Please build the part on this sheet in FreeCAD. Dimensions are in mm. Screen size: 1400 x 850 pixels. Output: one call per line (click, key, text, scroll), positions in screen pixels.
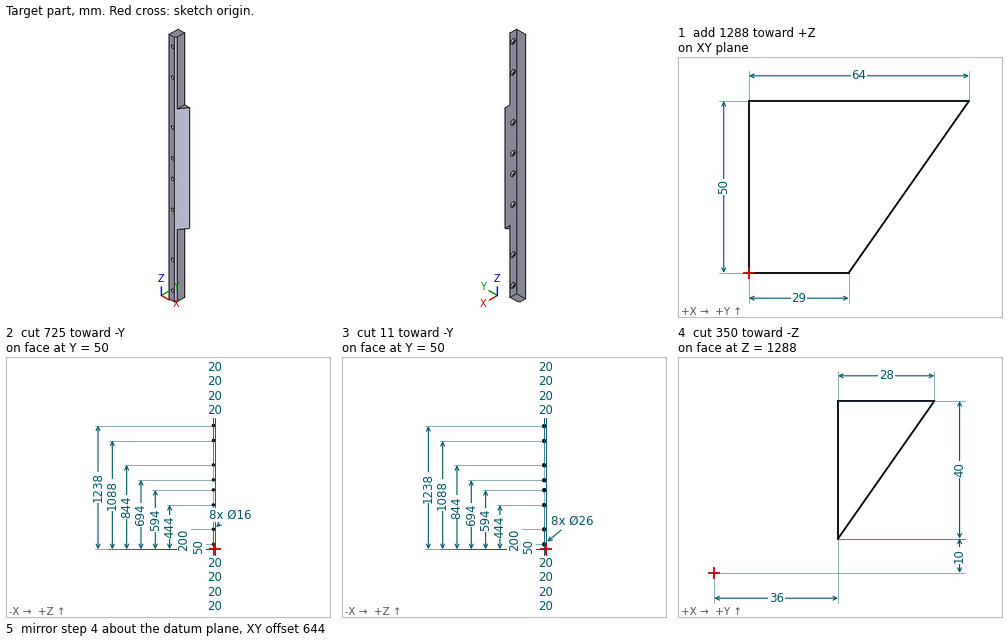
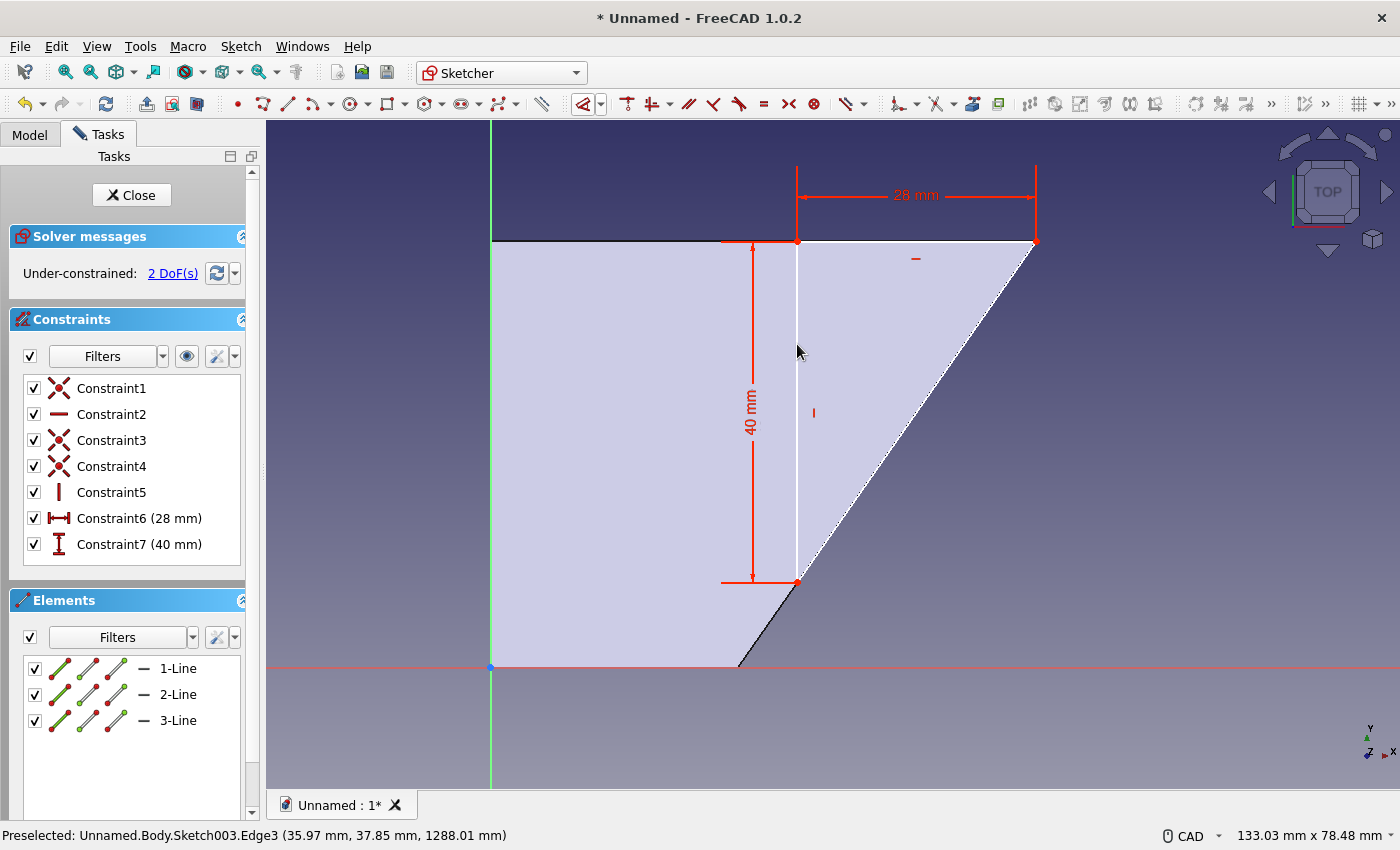
click(797, 583)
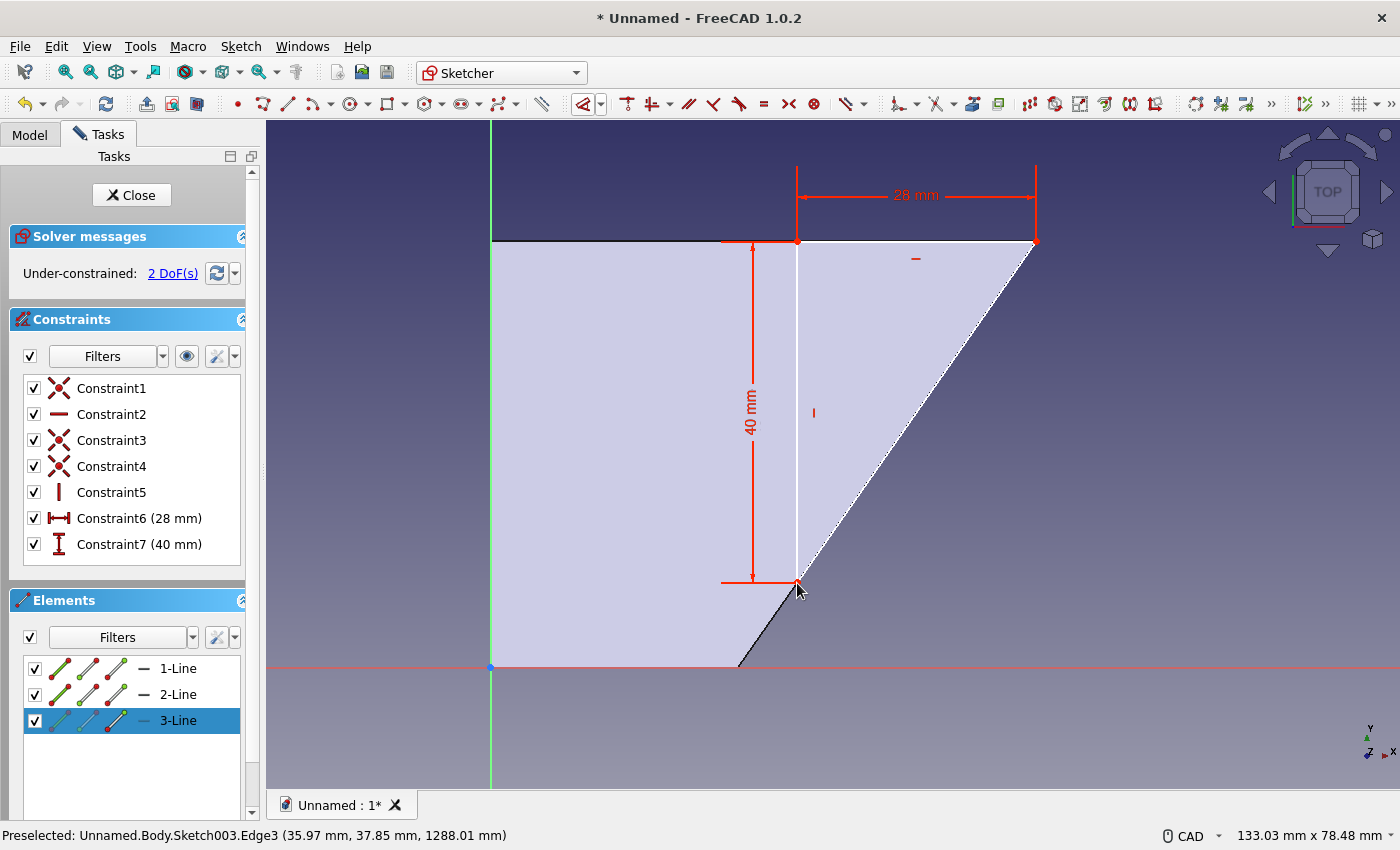
key(l)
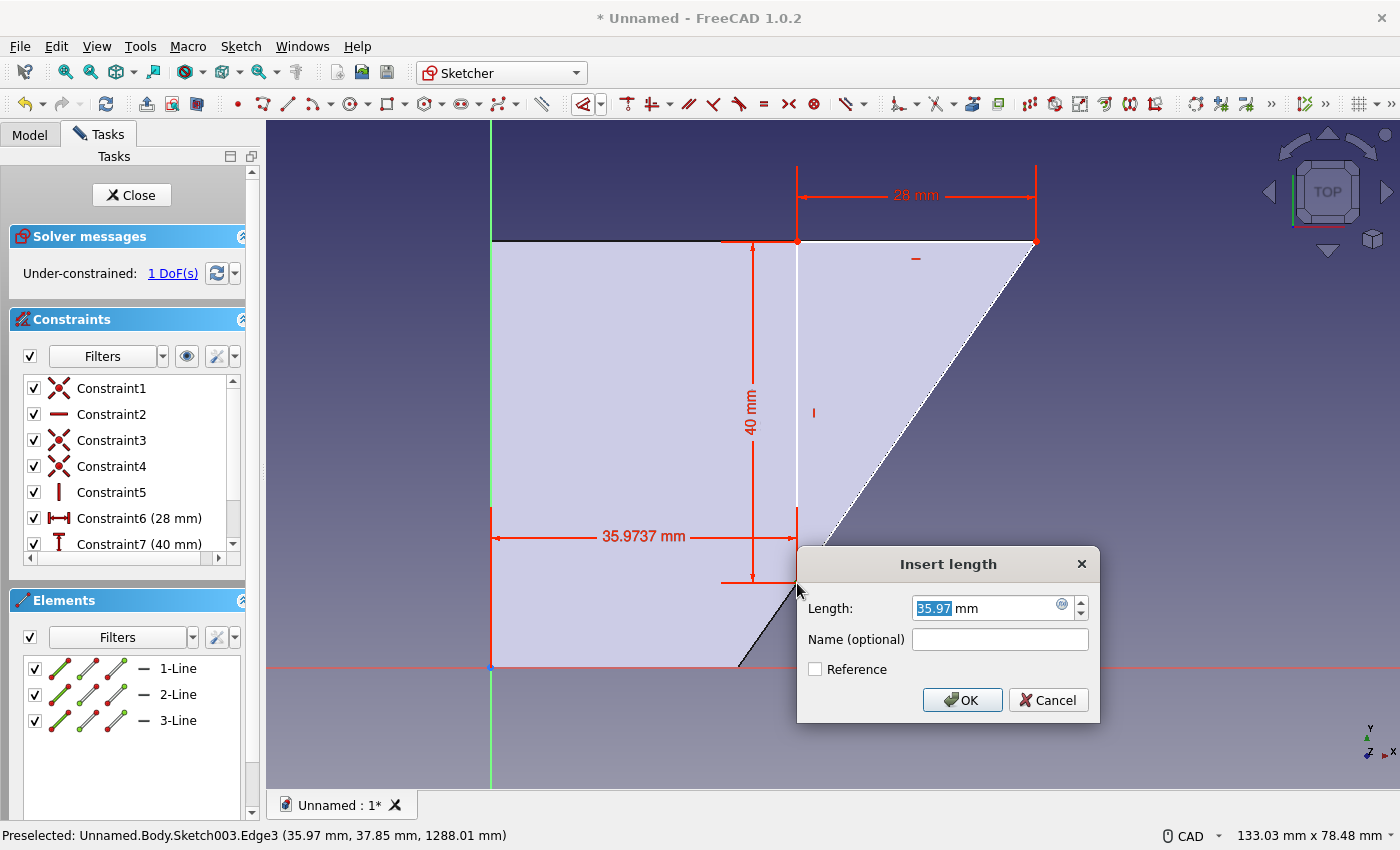
text(36)
key(Return)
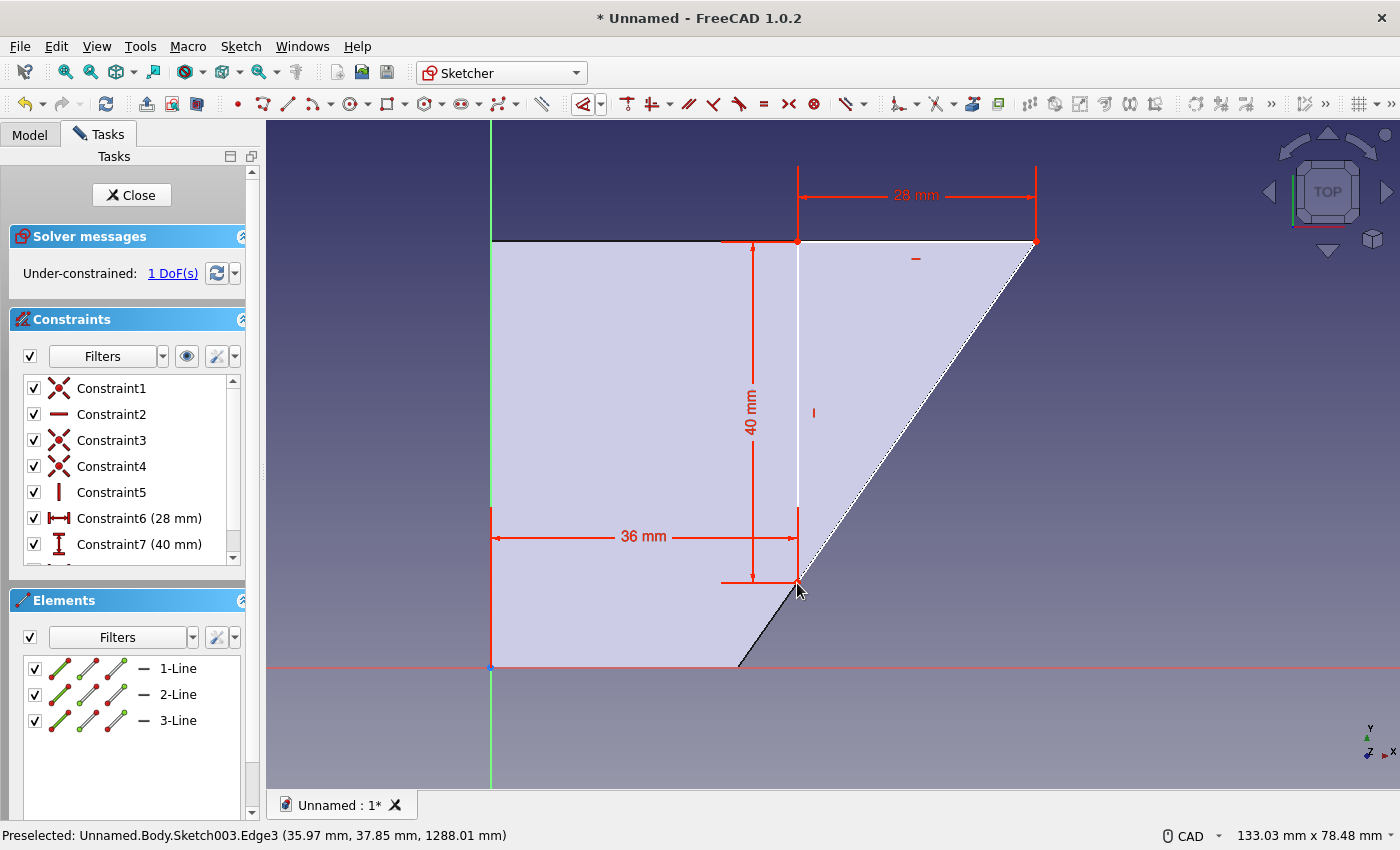
click(798, 583)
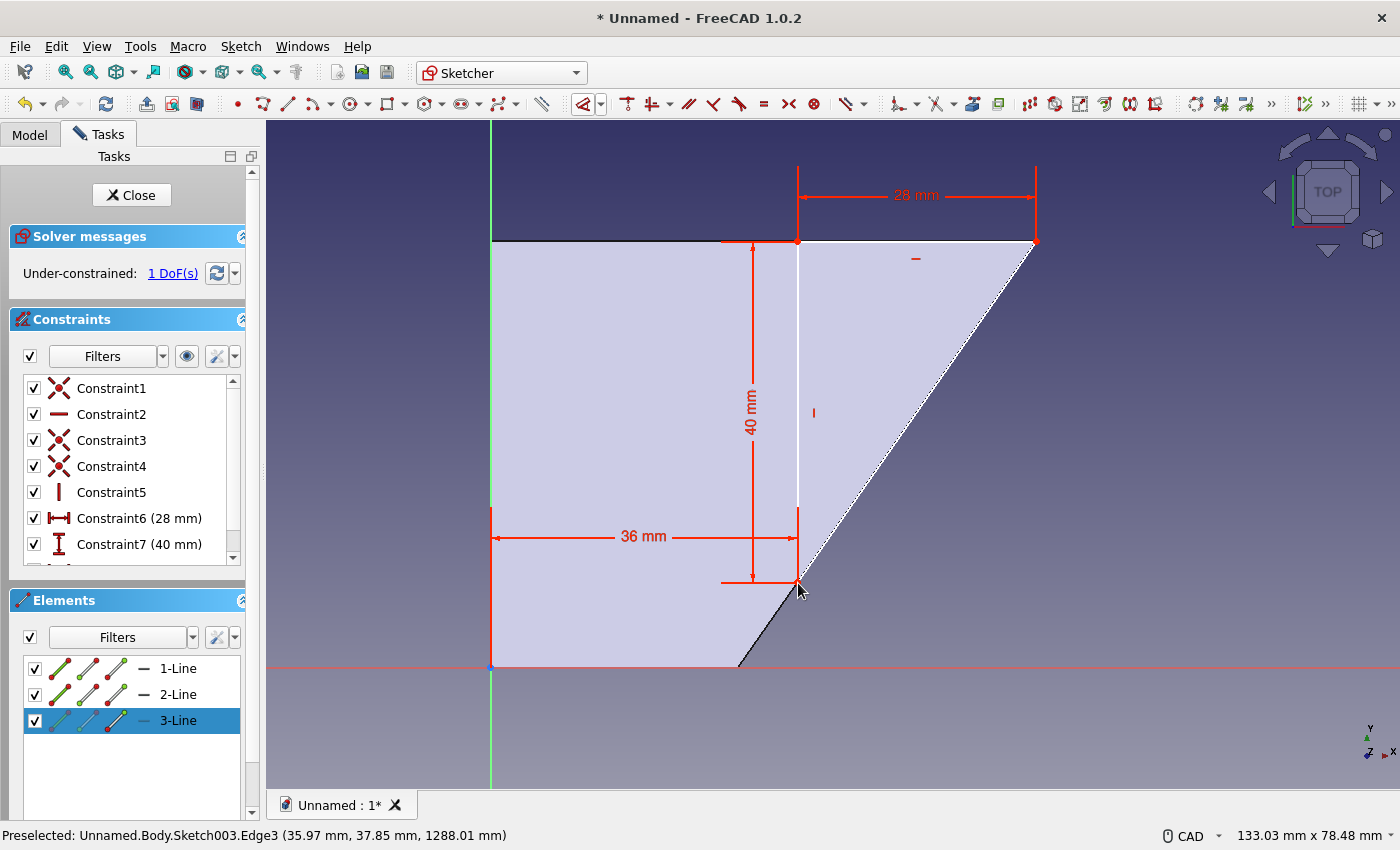
key(i)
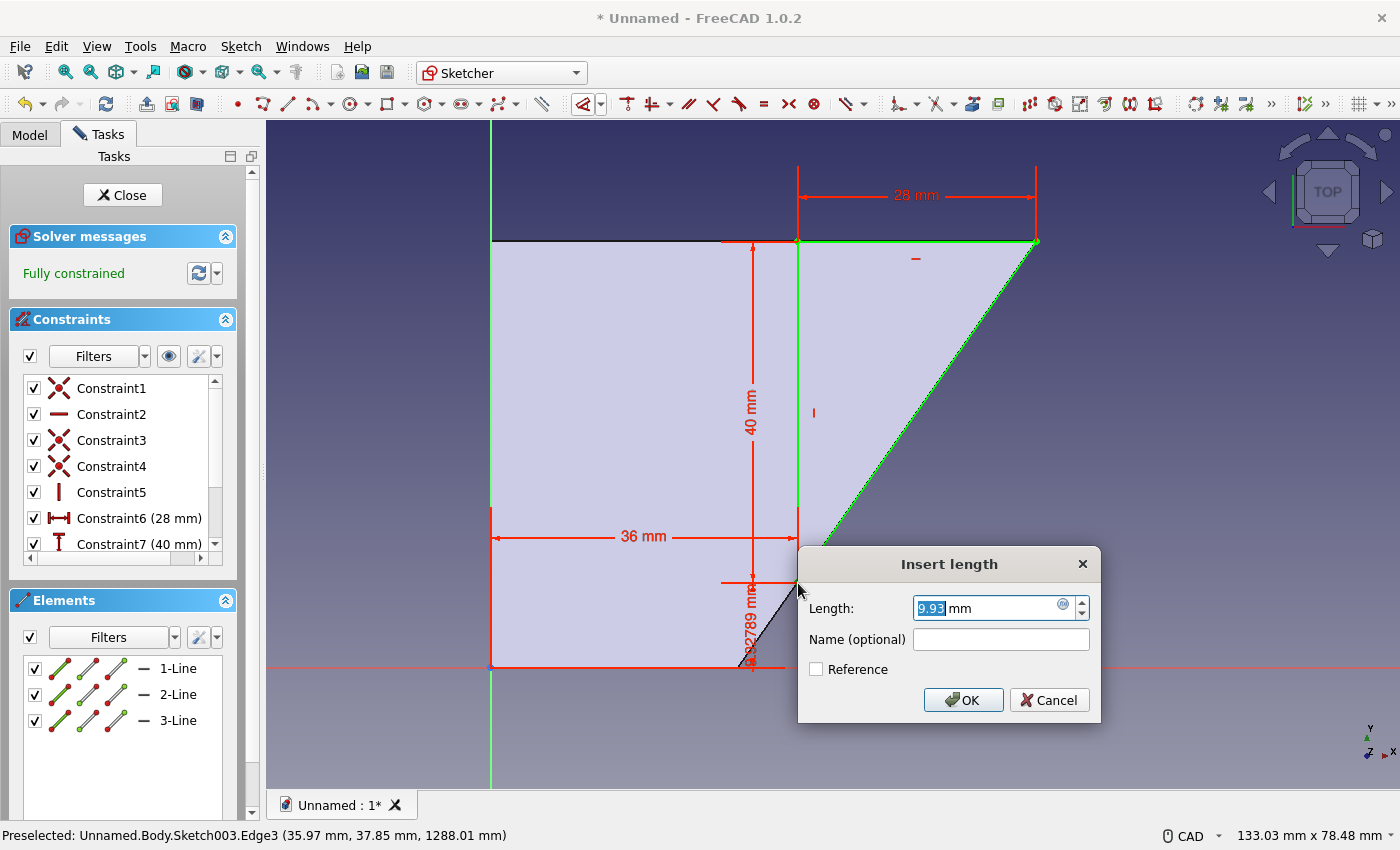
text(10)
key(Return)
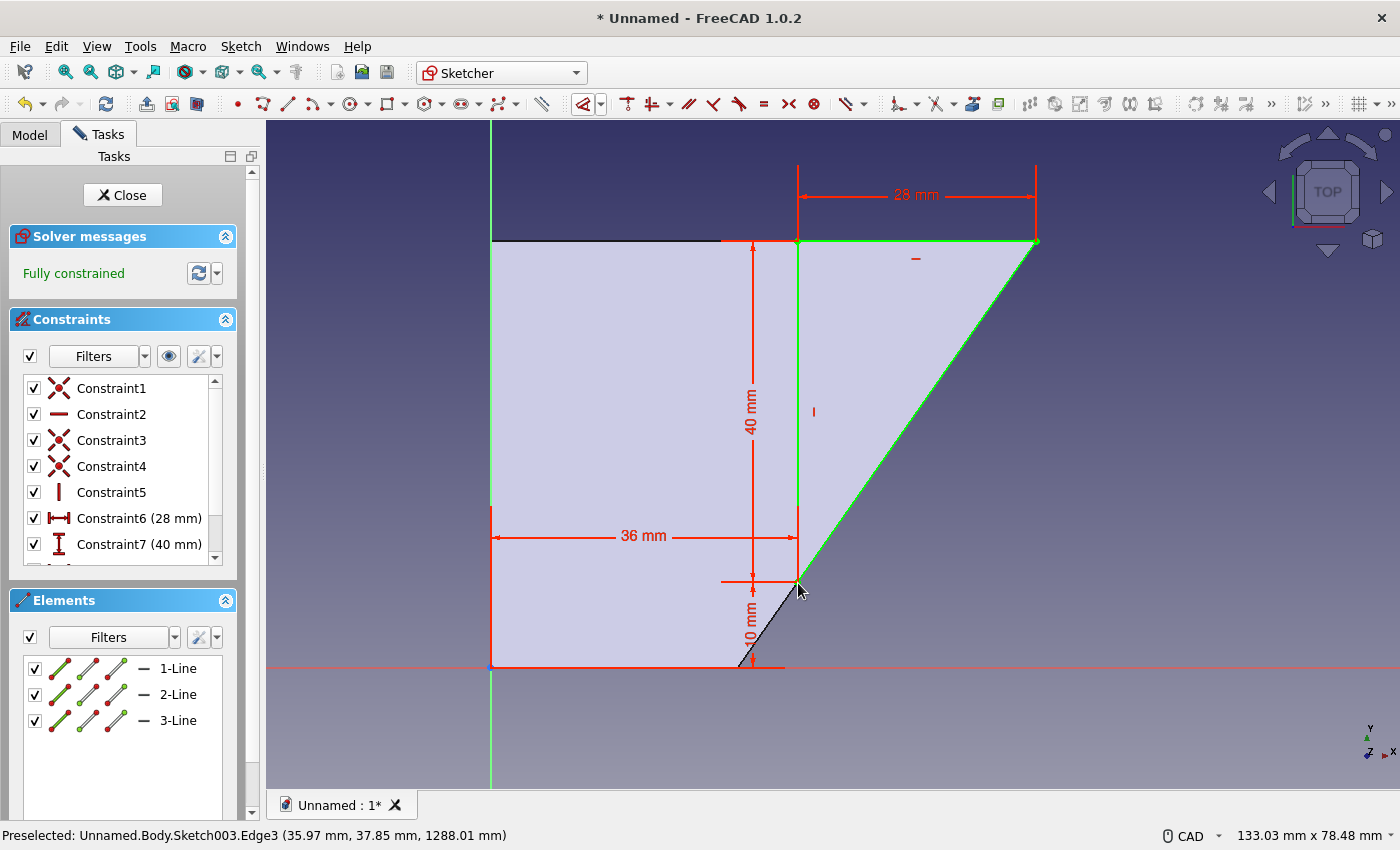
click(123, 195)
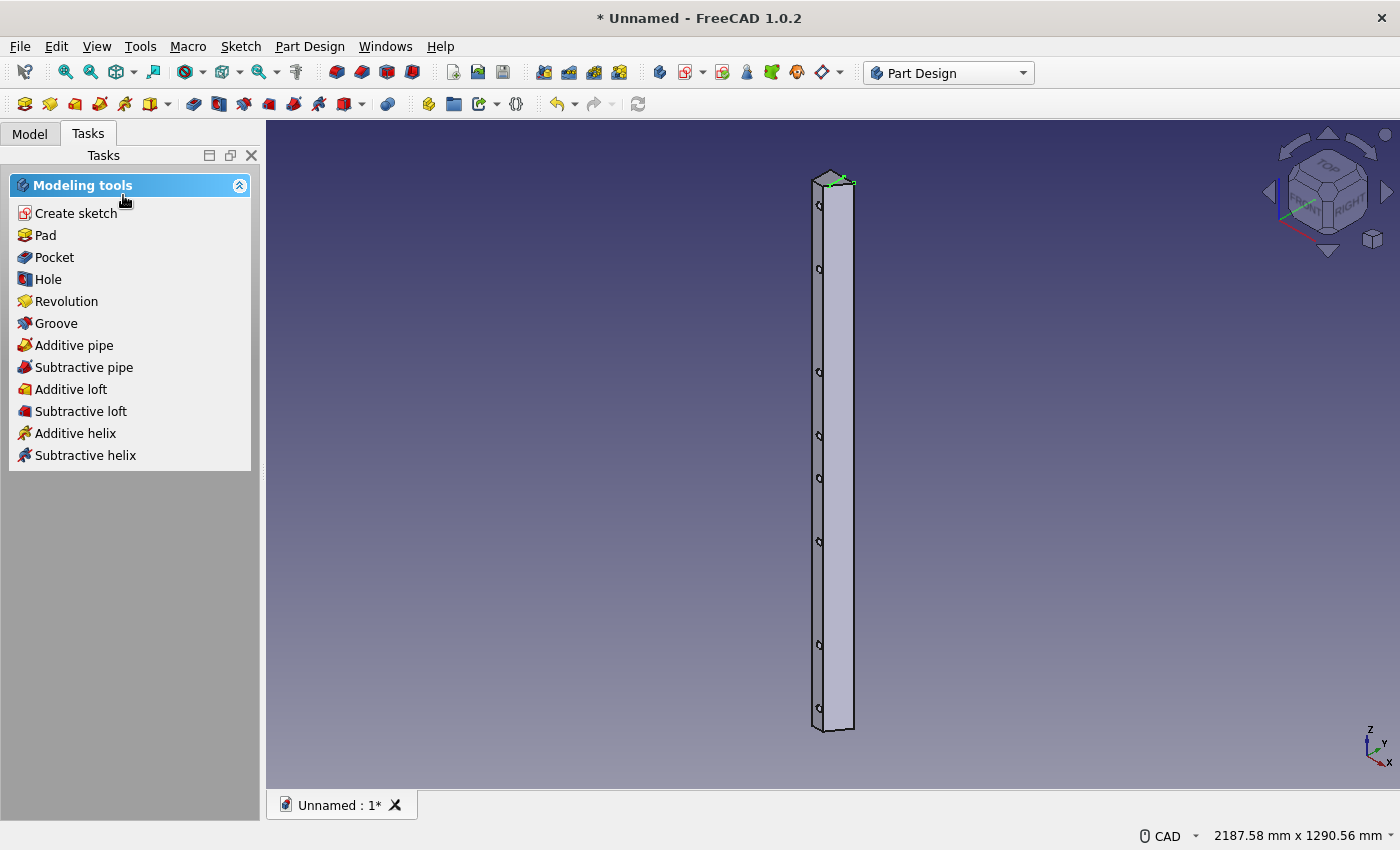
click(194, 104)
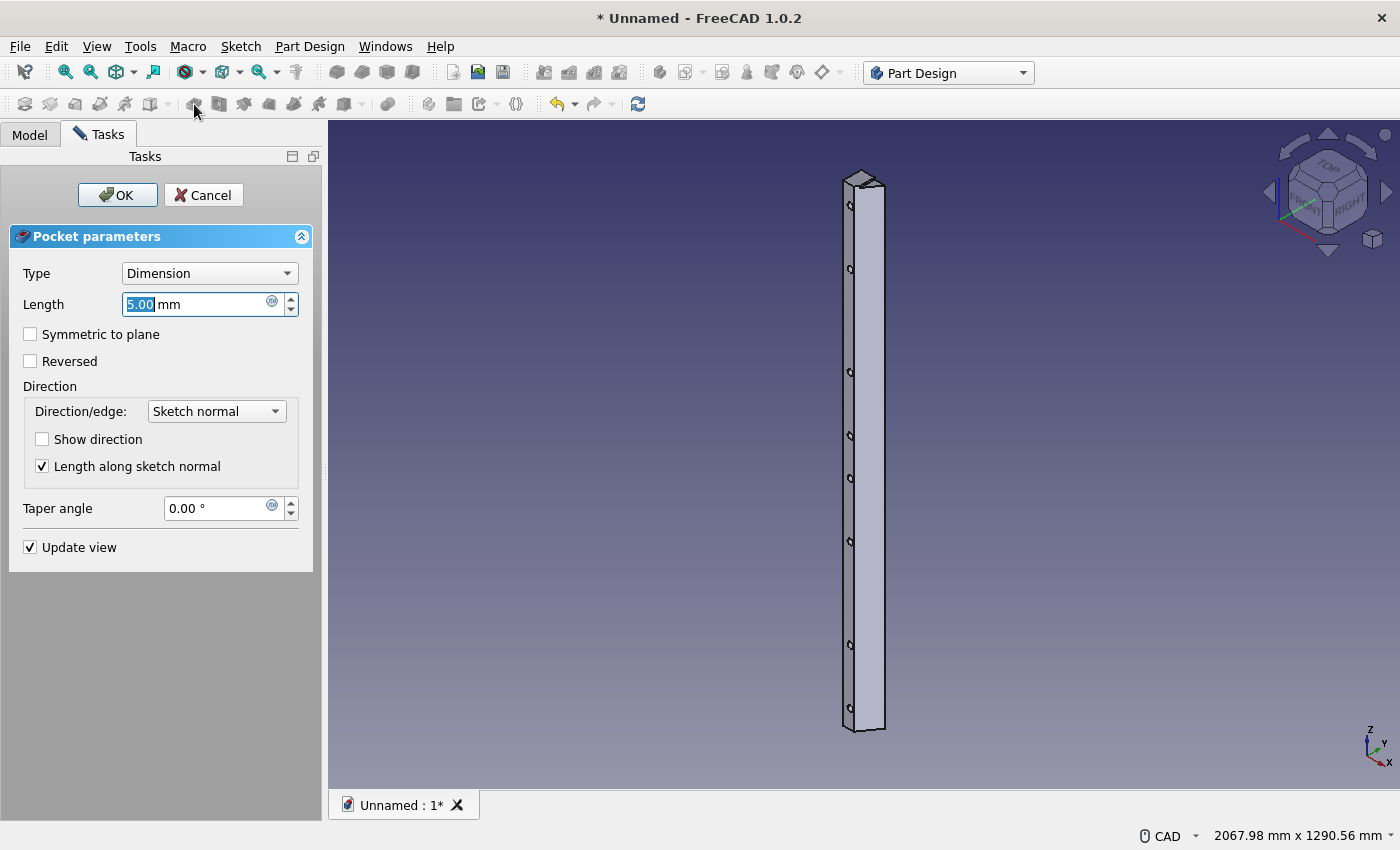
text(350)
key(Tab)